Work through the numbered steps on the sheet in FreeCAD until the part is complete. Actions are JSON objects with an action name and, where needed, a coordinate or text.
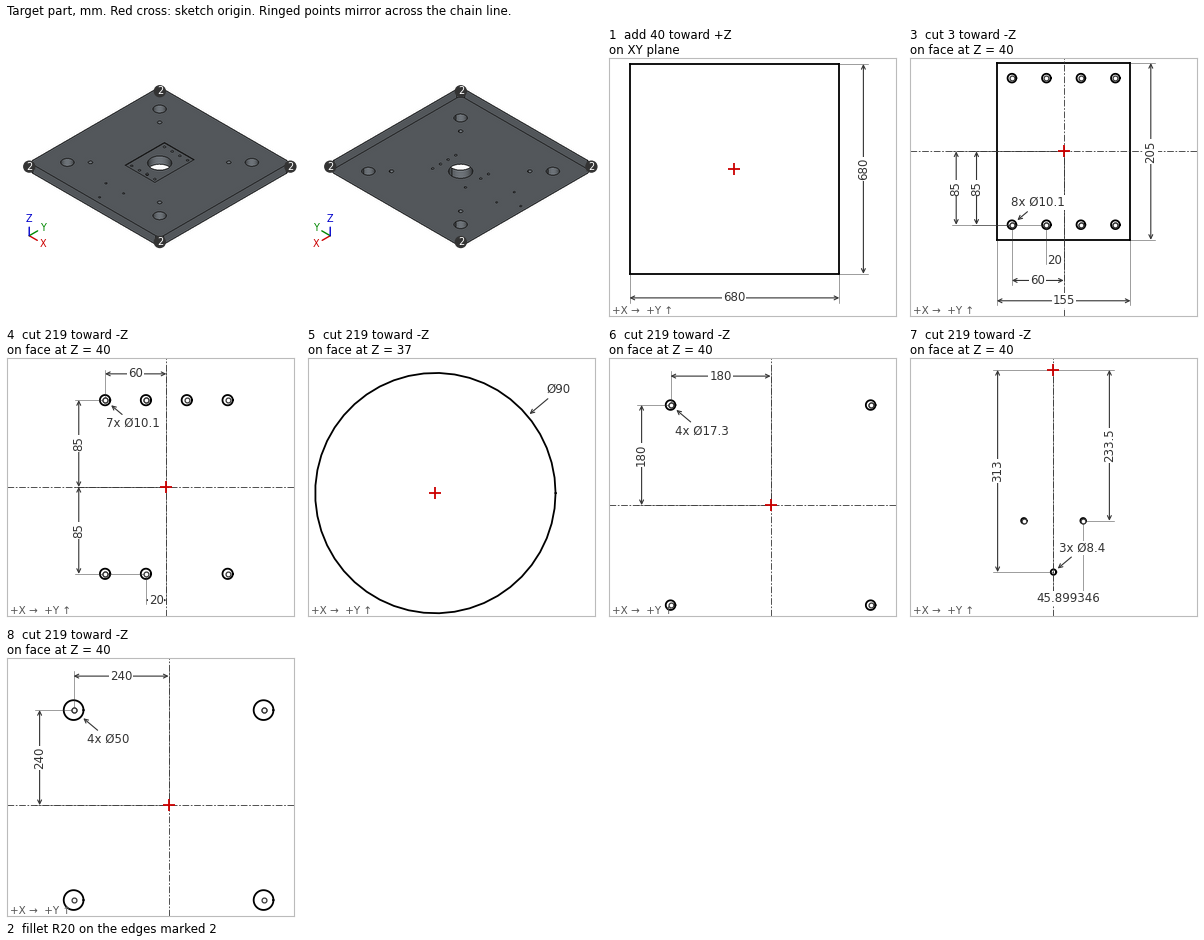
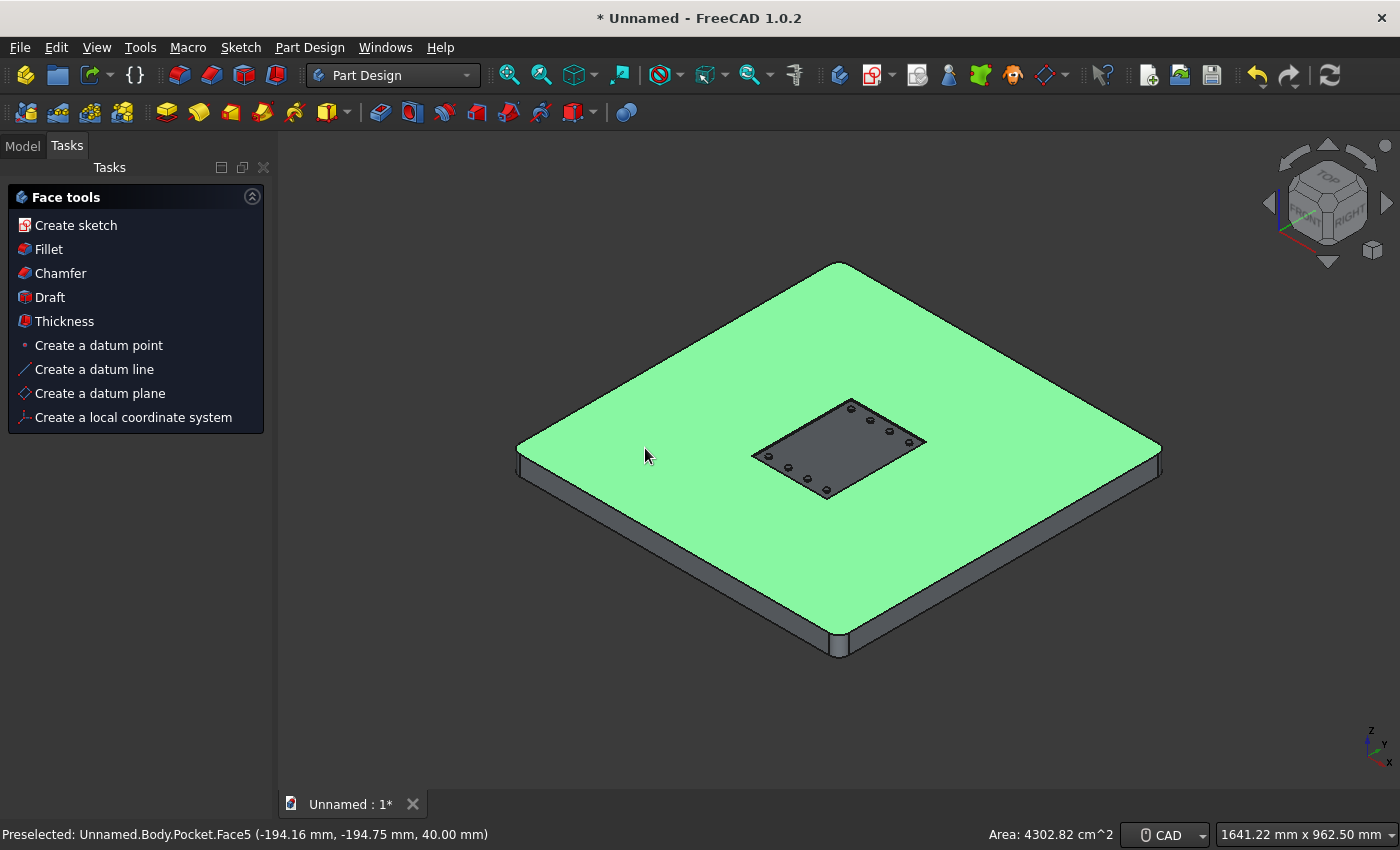
{"action": "left_click", "coordinate": [872, 76]}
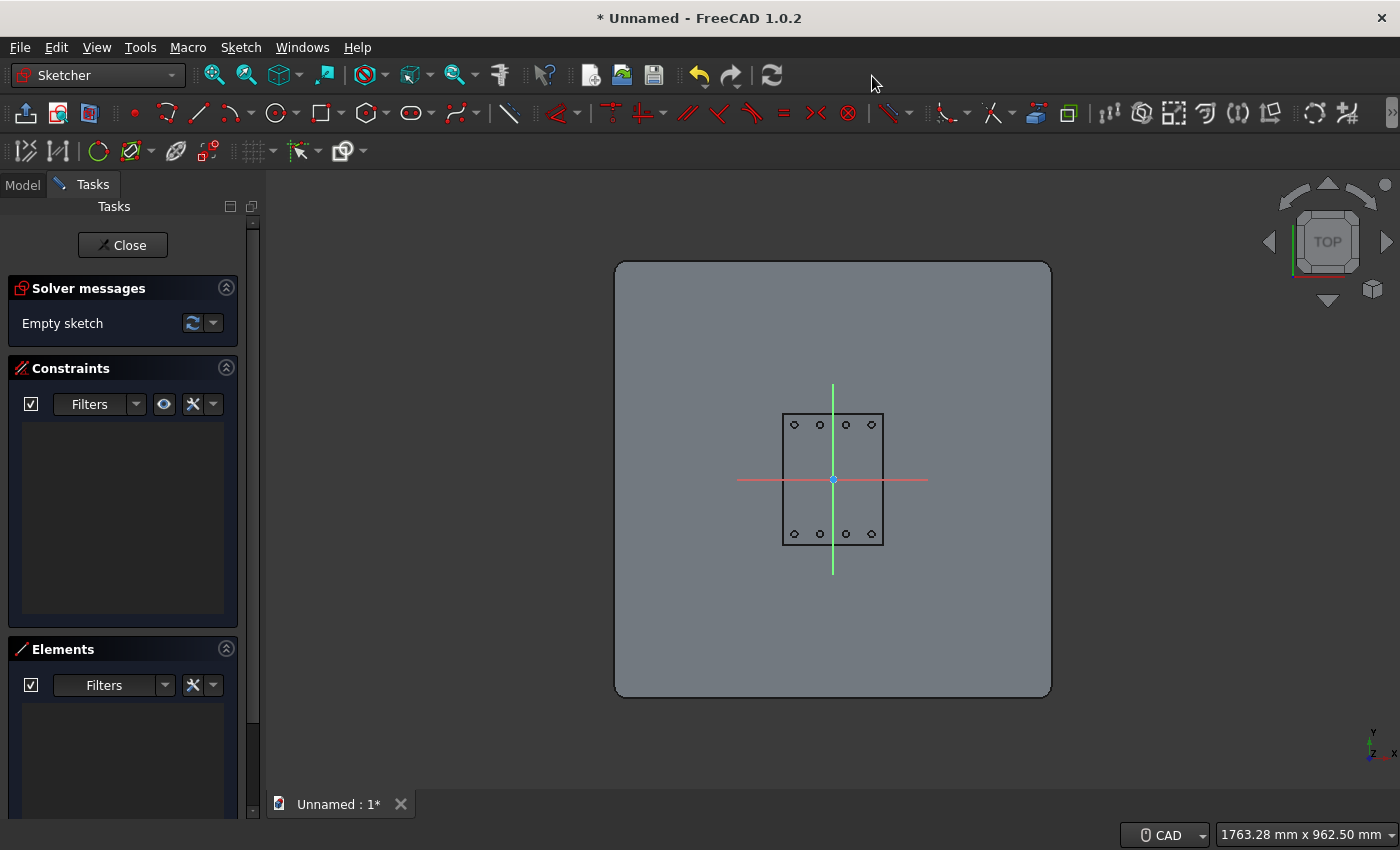
{"action": "scroll", "coordinate": [863, 479], "scroll_direction": "up", "scroll_amount": 6}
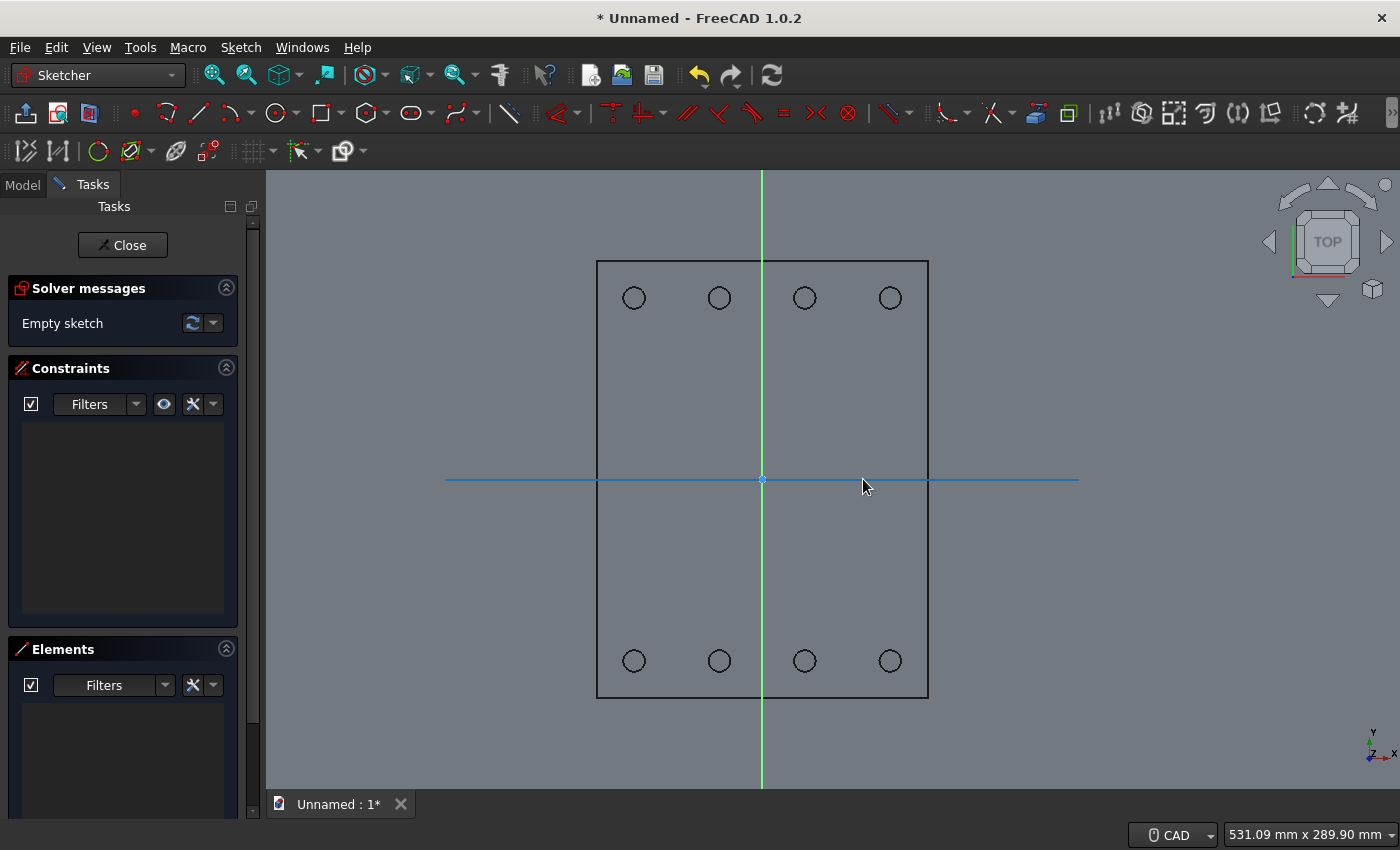
{"action": "left_click", "coordinate": [276, 114]}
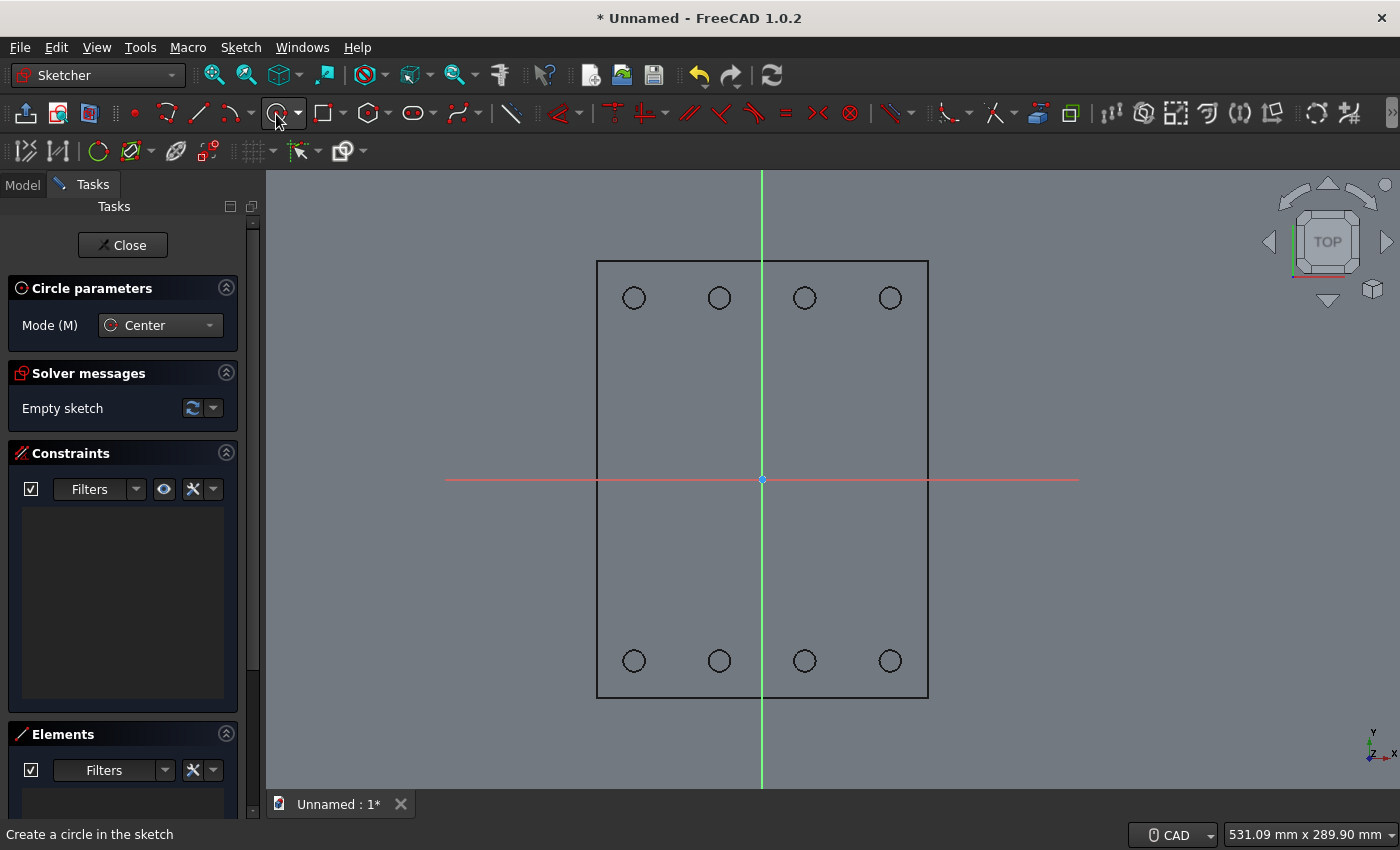
{"action": "scroll", "coordinate": [634, 298], "scroll_direction": "up", "scroll_amount": 4}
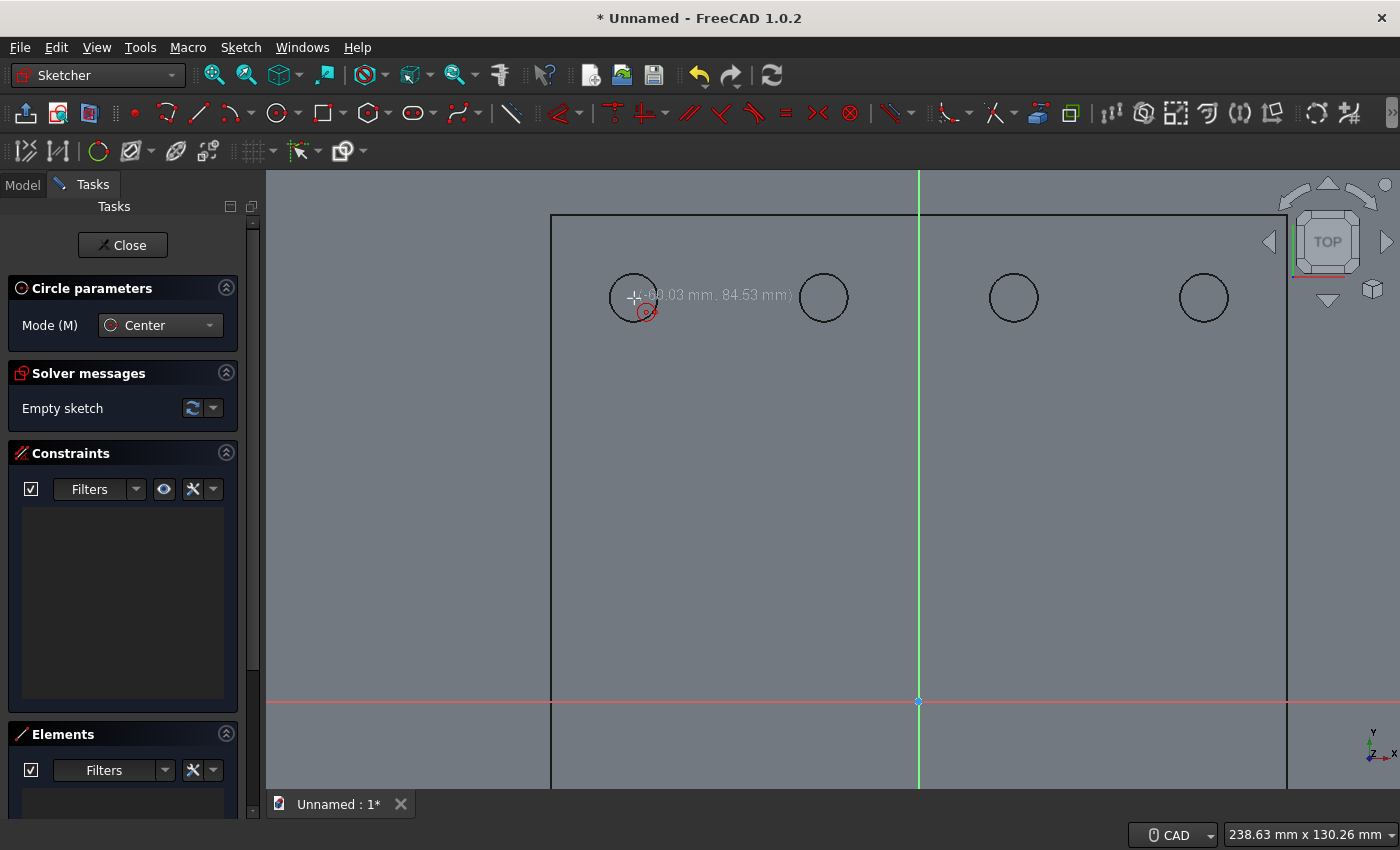
{"action": "left_click", "coordinate": [634, 298]}
{"action": "left_click", "coordinate": [651, 281]}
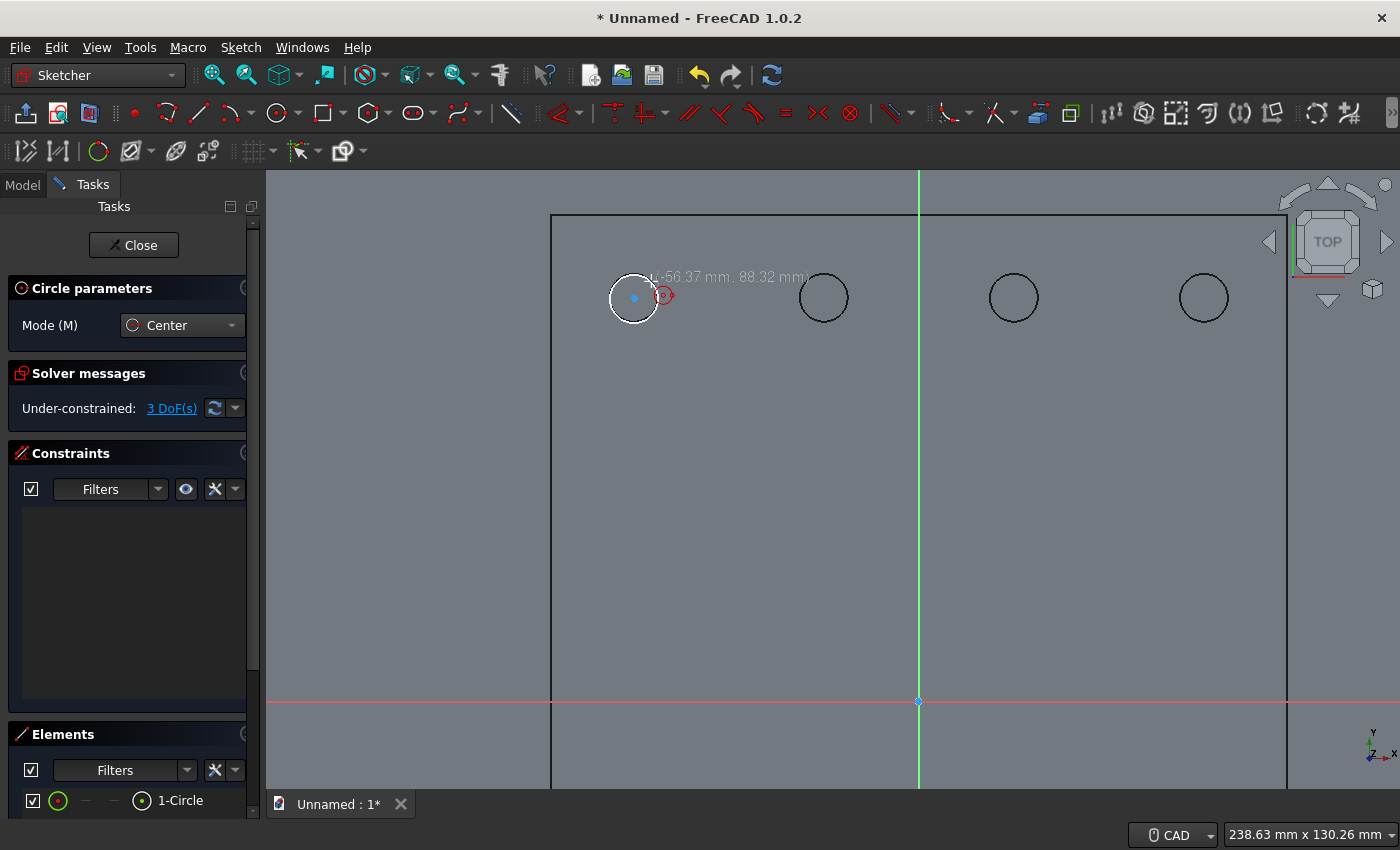
{"action": "scroll", "coordinate": [639, 298], "scroll_direction": "down", "scroll_amount": 4}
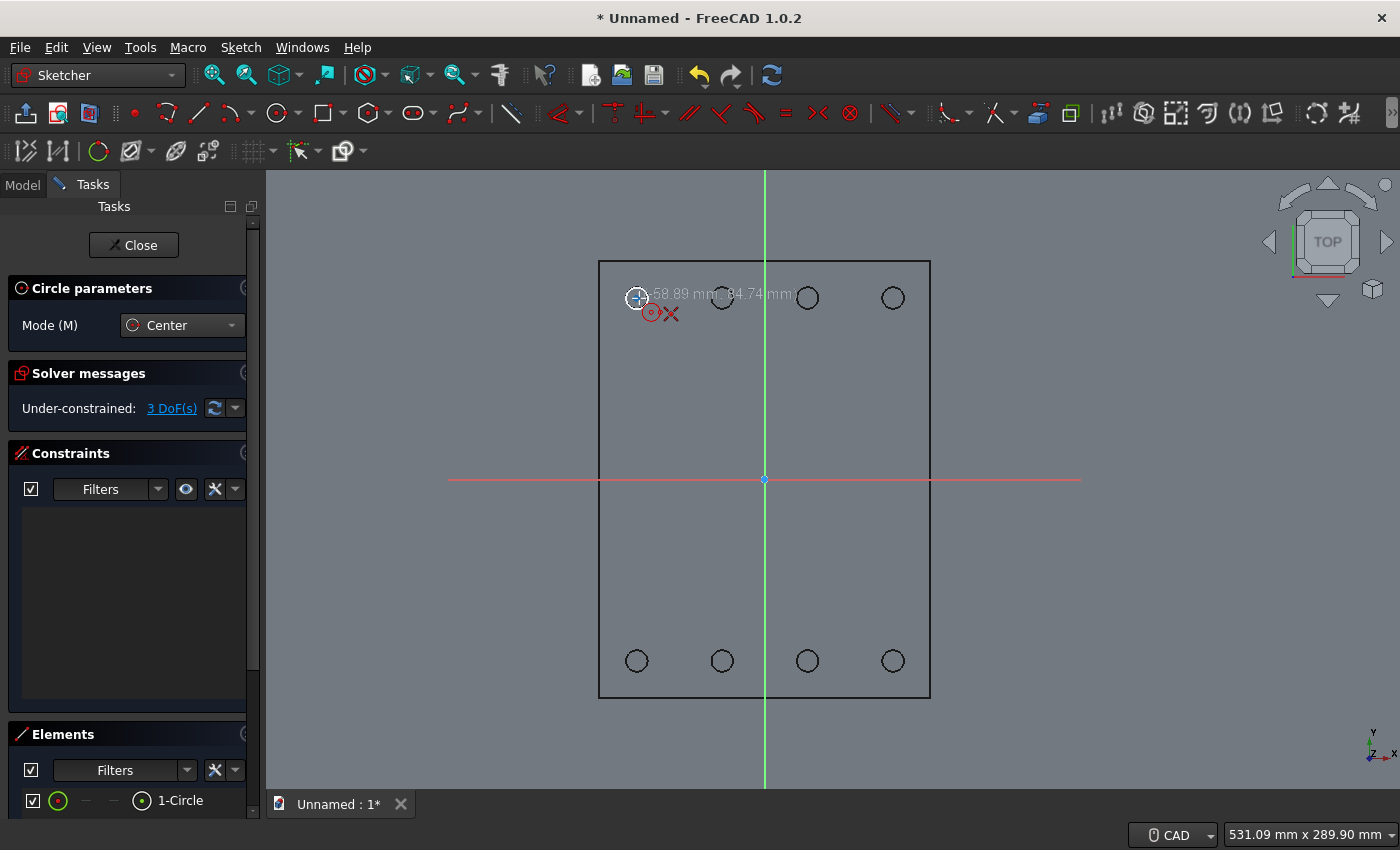
{"action": "scroll", "coordinate": [637, 661], "scroll_direction": "up", "scroll_amount": 4}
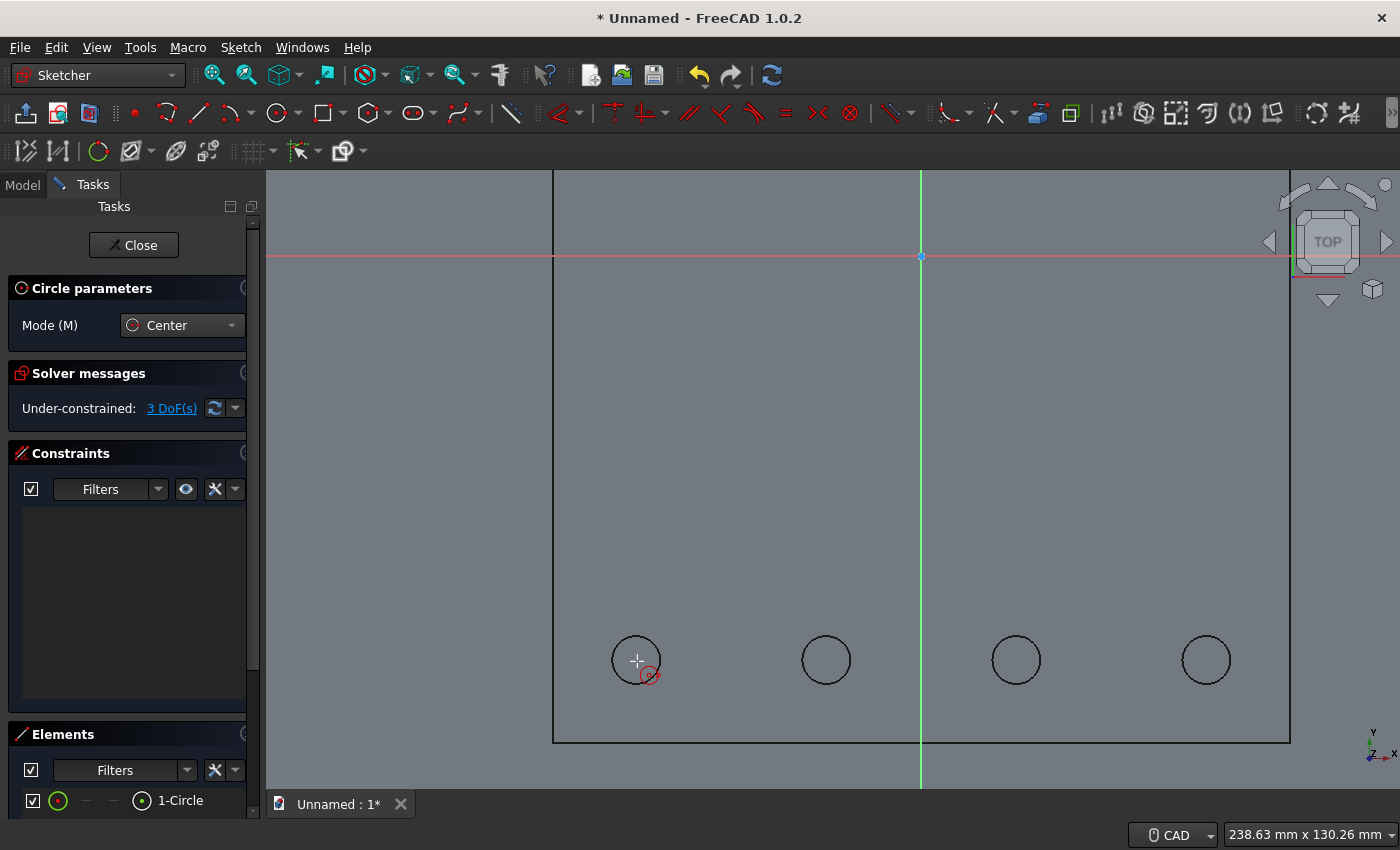
{"action": "left_click", "coordinate": [636, 660]}
{"action": "left_click", "coordinate": [653, 643]}